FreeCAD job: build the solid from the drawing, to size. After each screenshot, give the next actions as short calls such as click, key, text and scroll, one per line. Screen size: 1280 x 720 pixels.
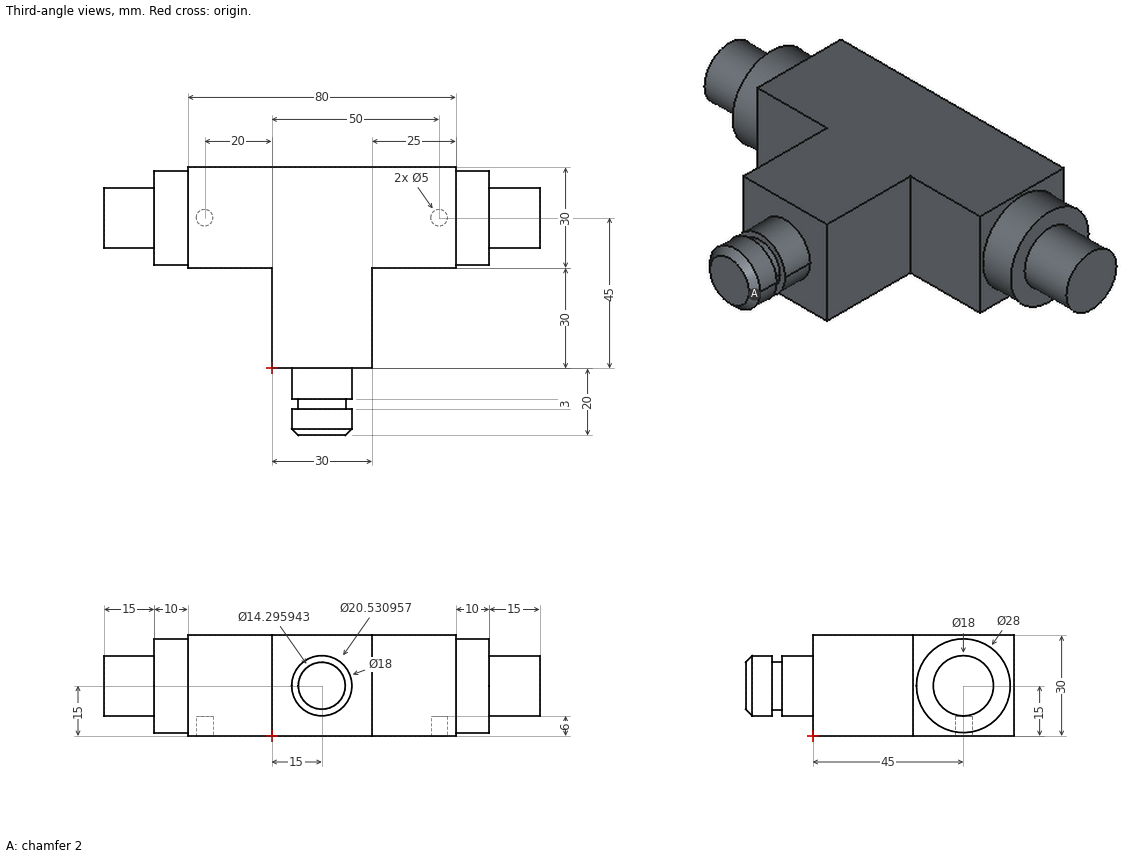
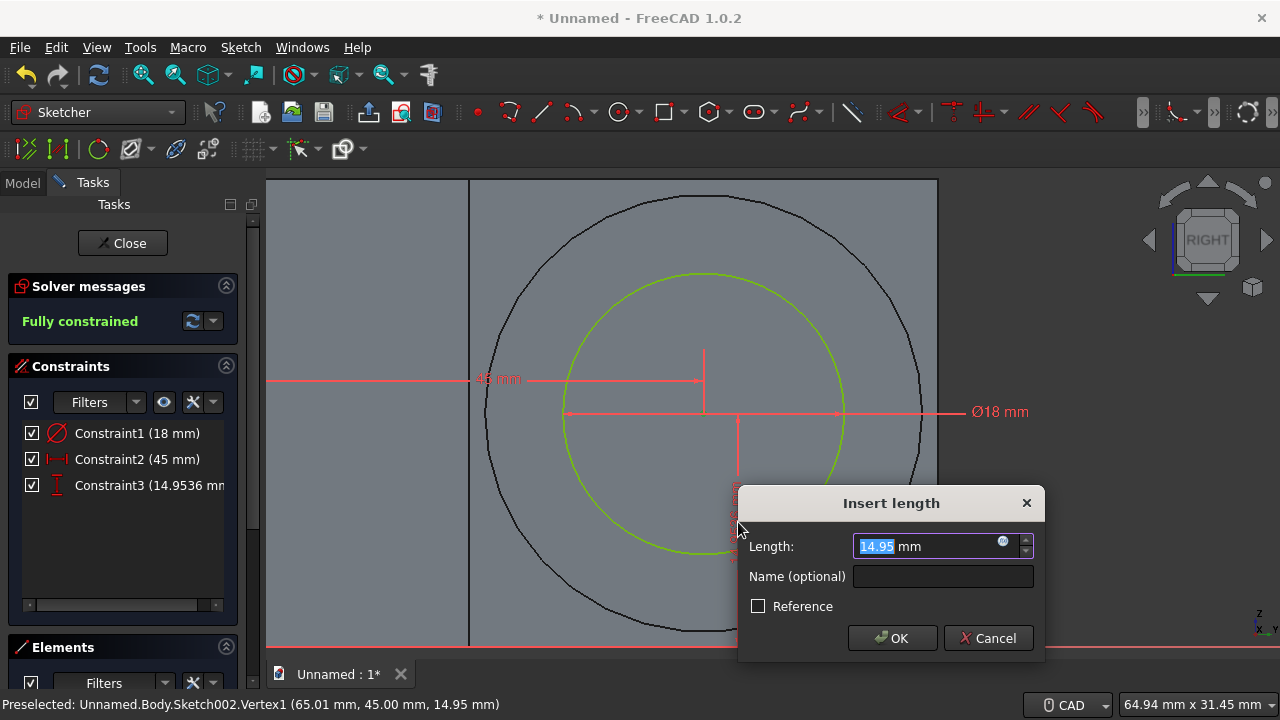
text(15)
key(Return)
key(Escape)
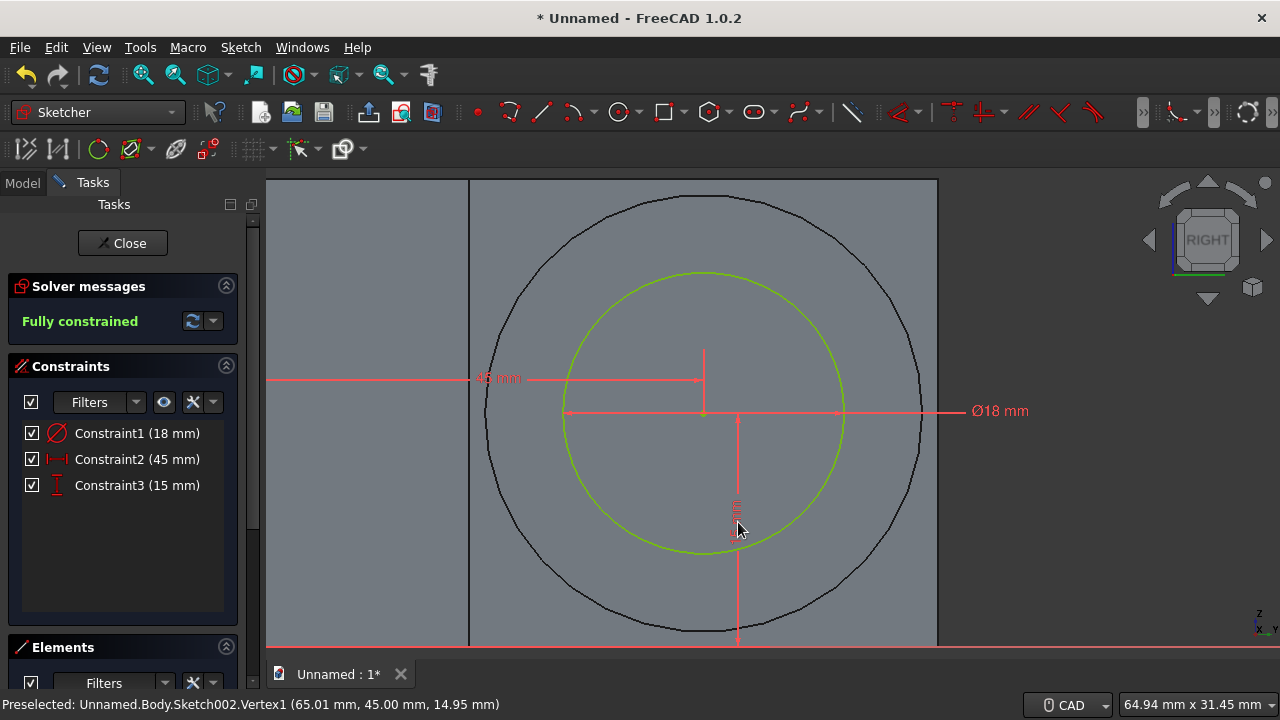
click(123, 243)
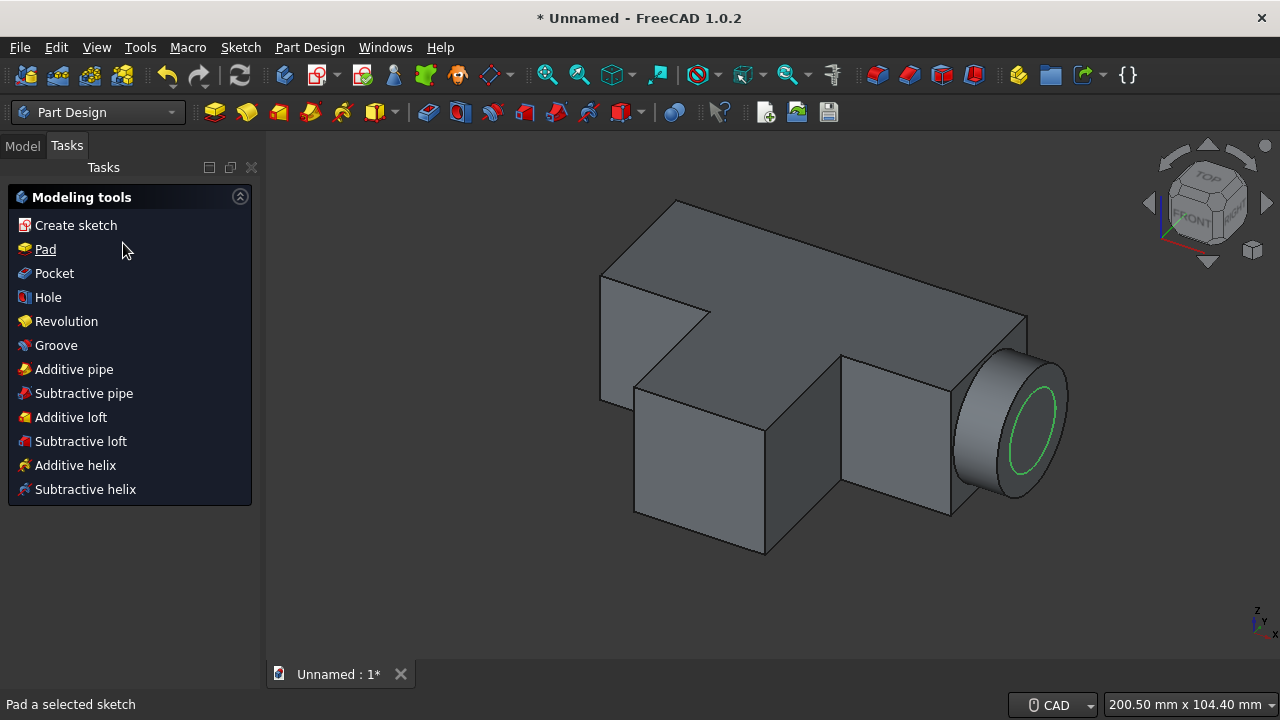
click(216, 112)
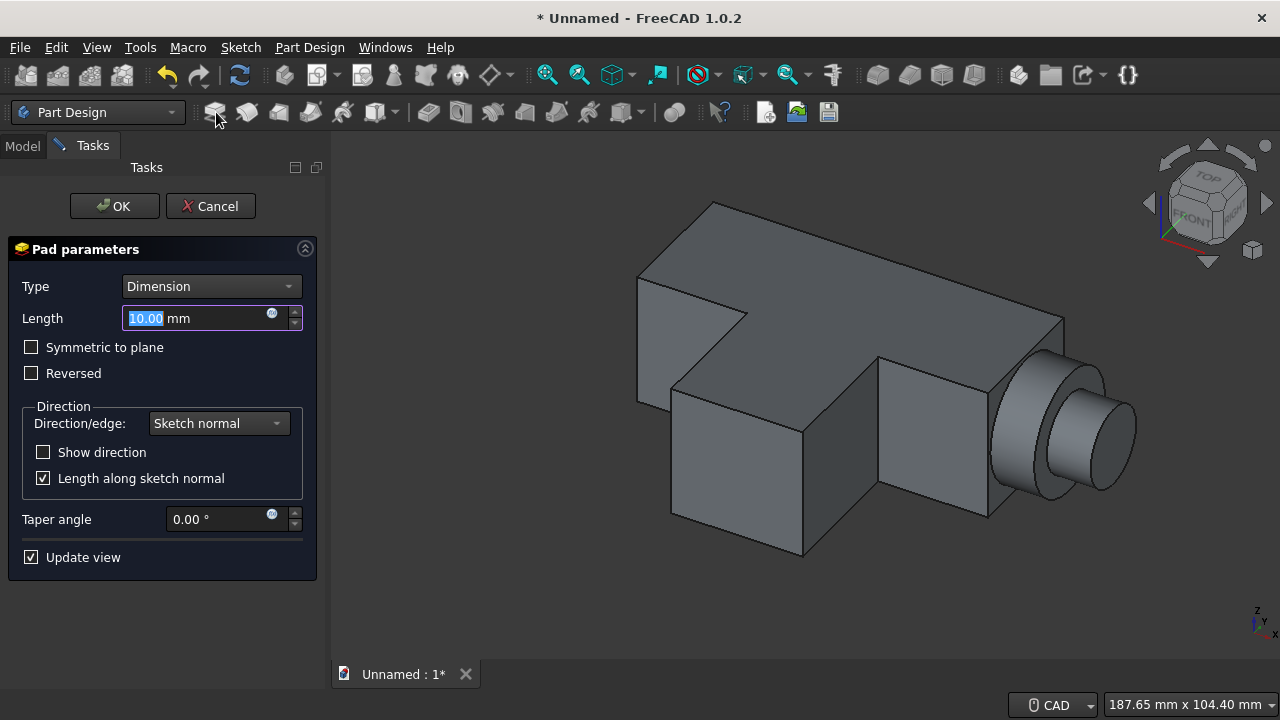
text(15)
key(Tab)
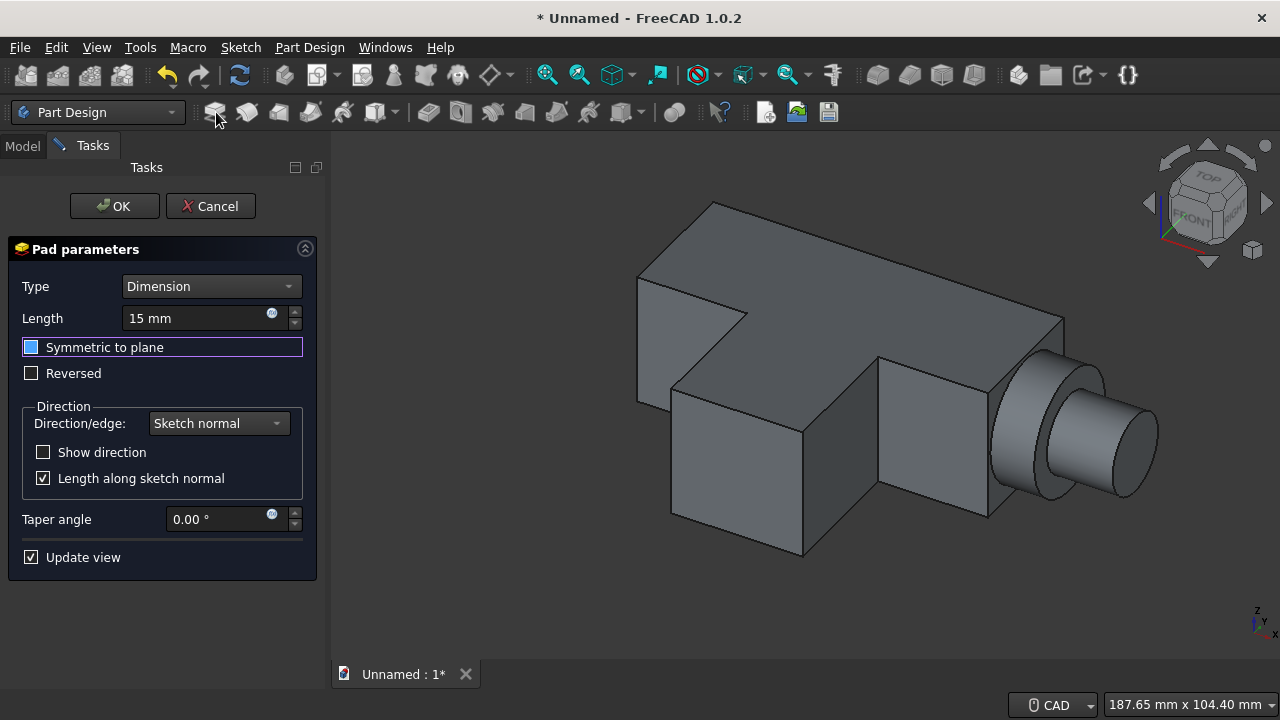
click(115, 206)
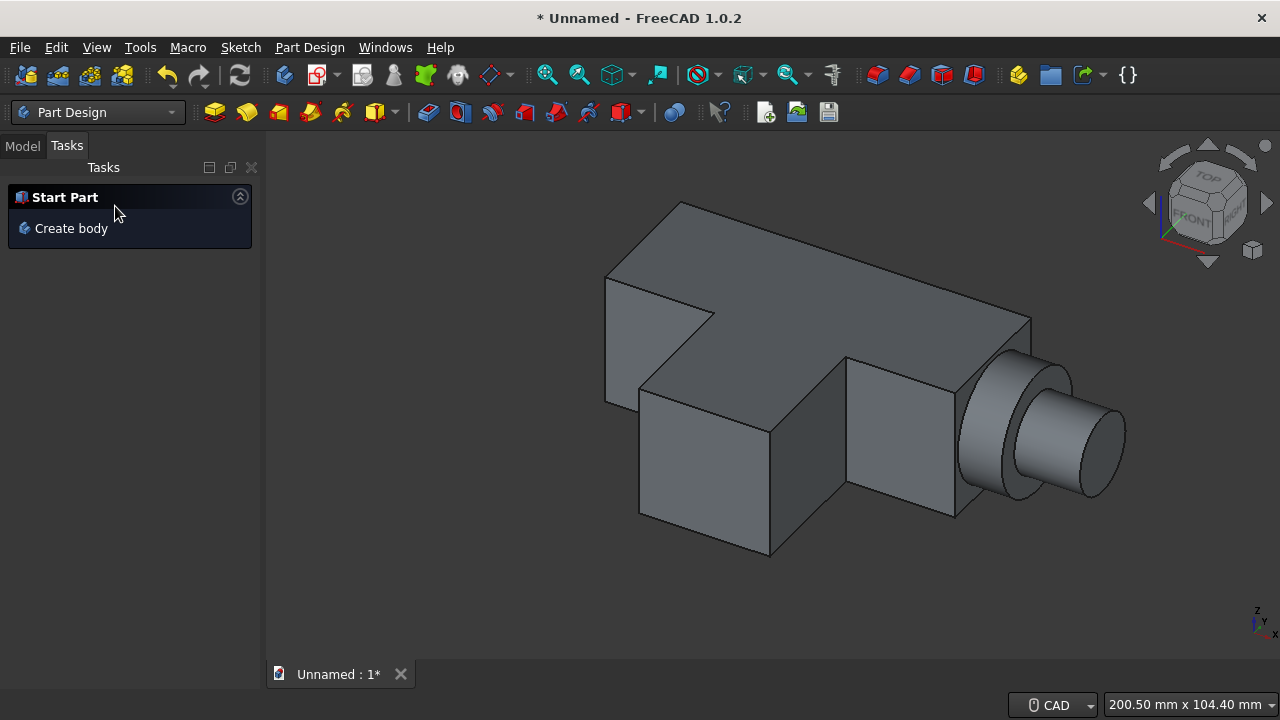
click(23, 145)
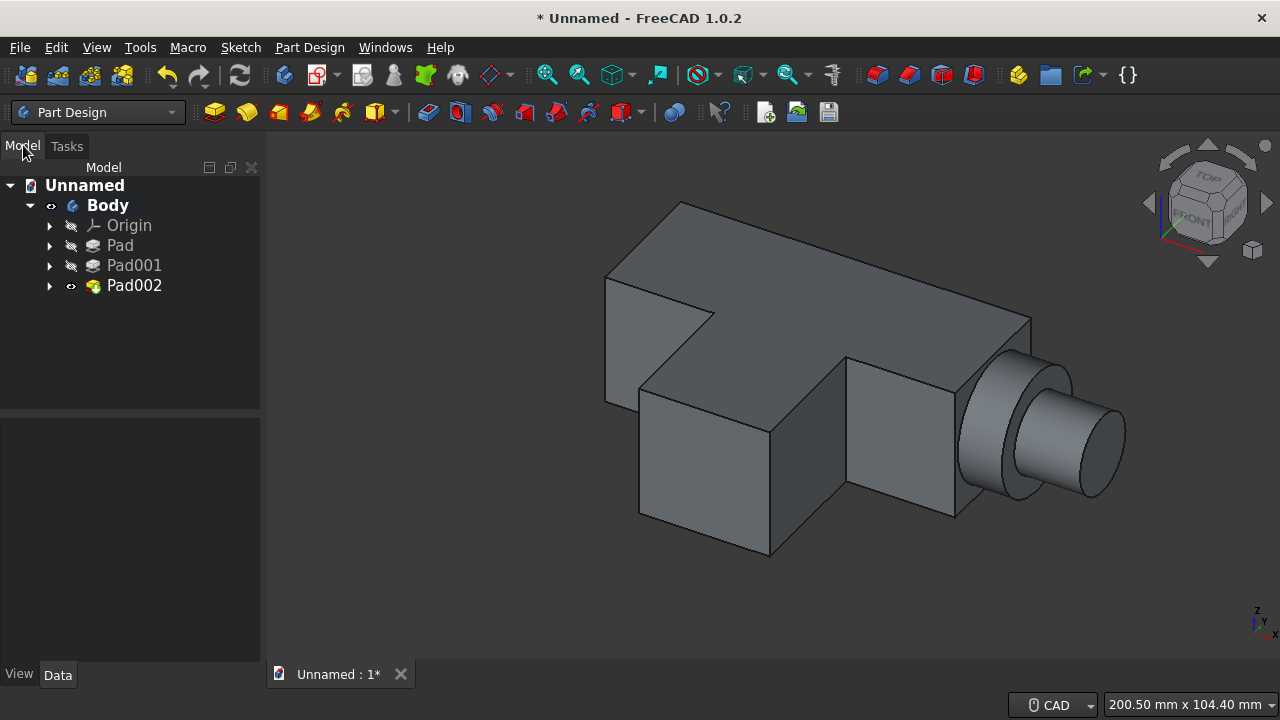
click(50, 226)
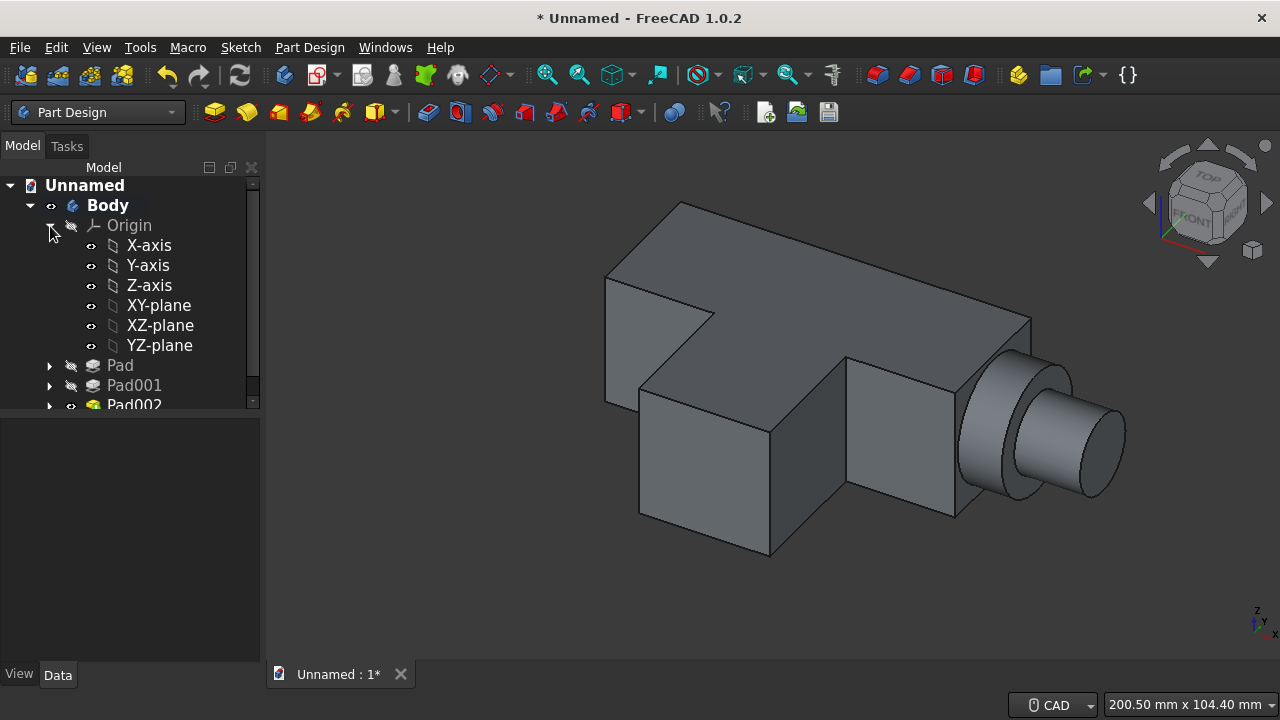
click(136, 346)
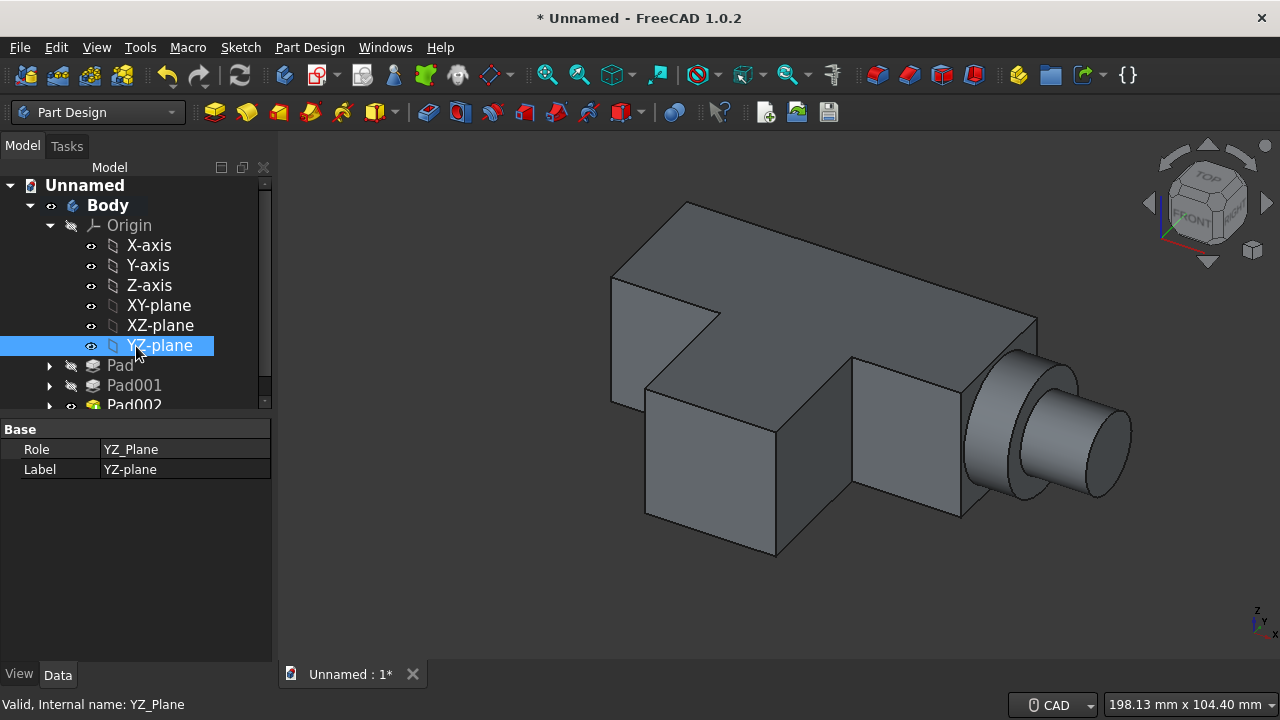
click(490, 76)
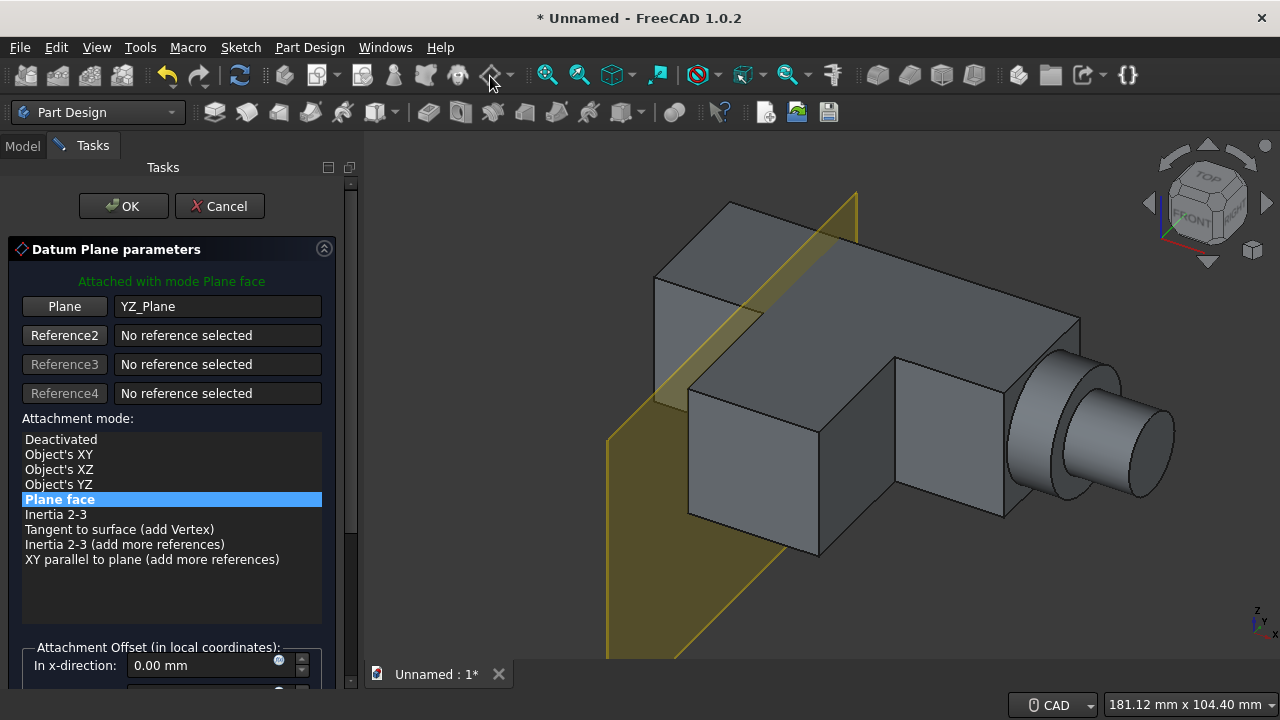
scroll(351, 432, down, 2)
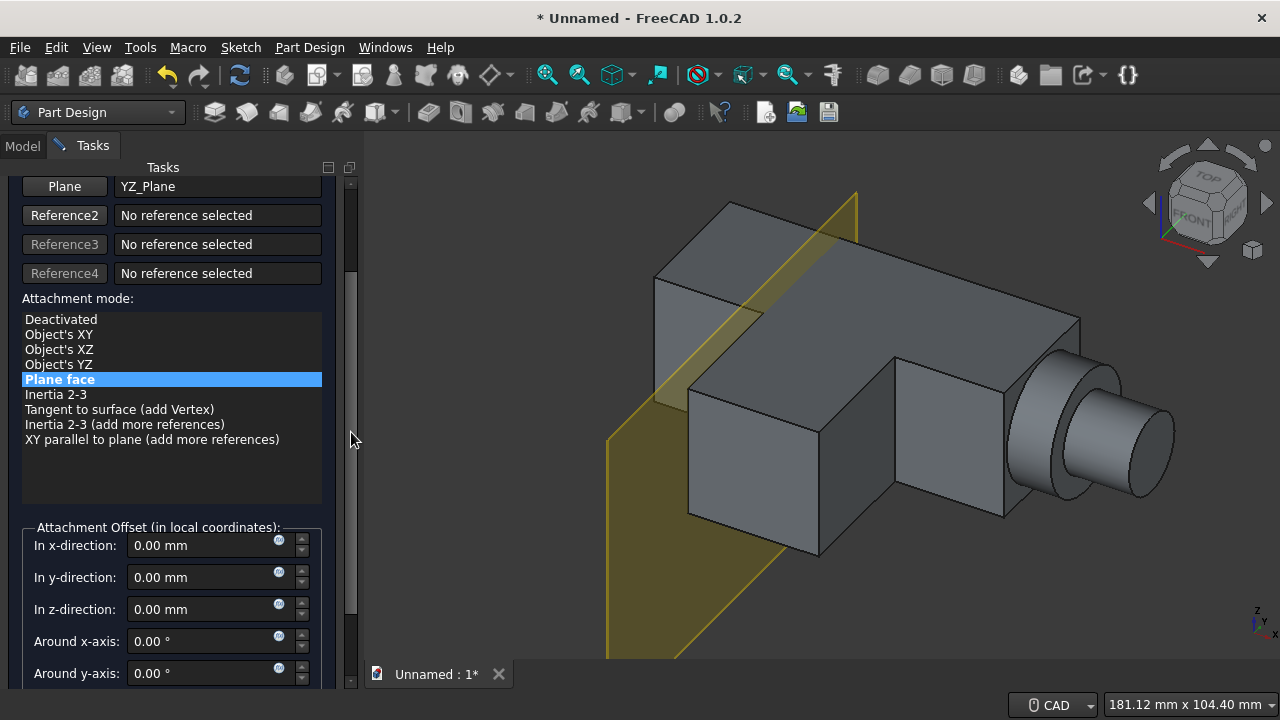
triple_click(210, 609)